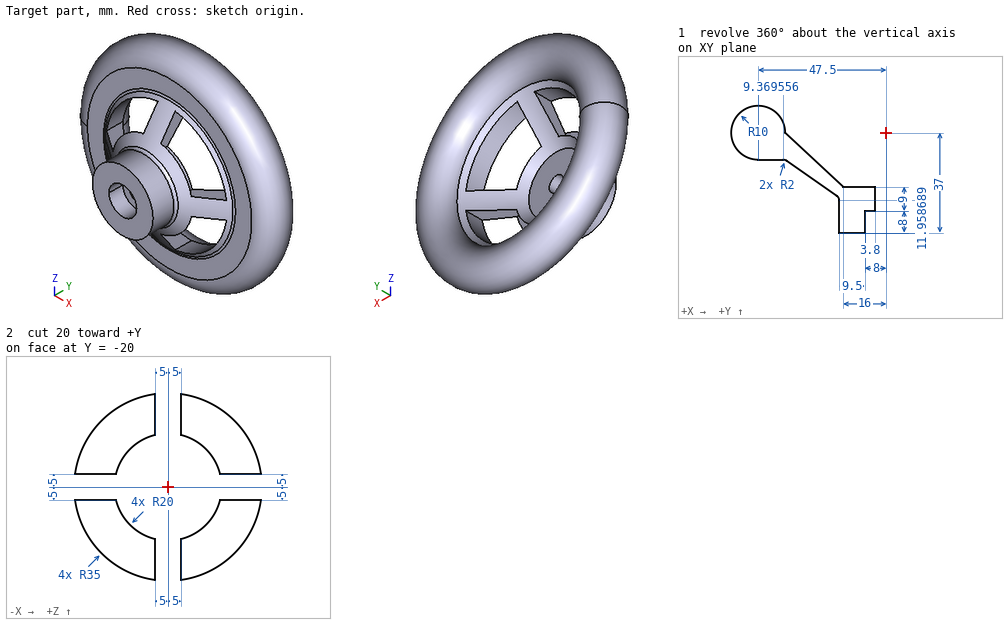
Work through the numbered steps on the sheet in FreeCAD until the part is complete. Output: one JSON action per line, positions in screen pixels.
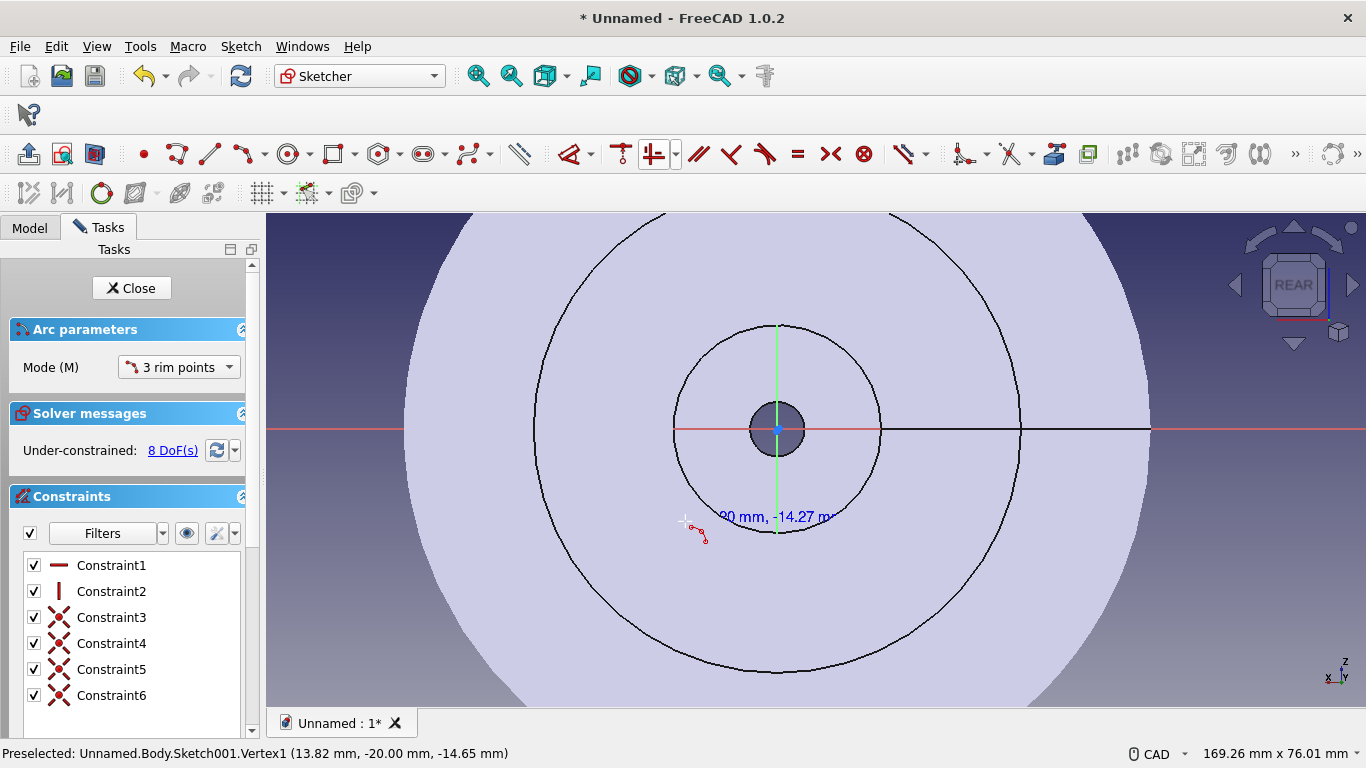
{"action": "left_click", "coordinate": [210, 154]}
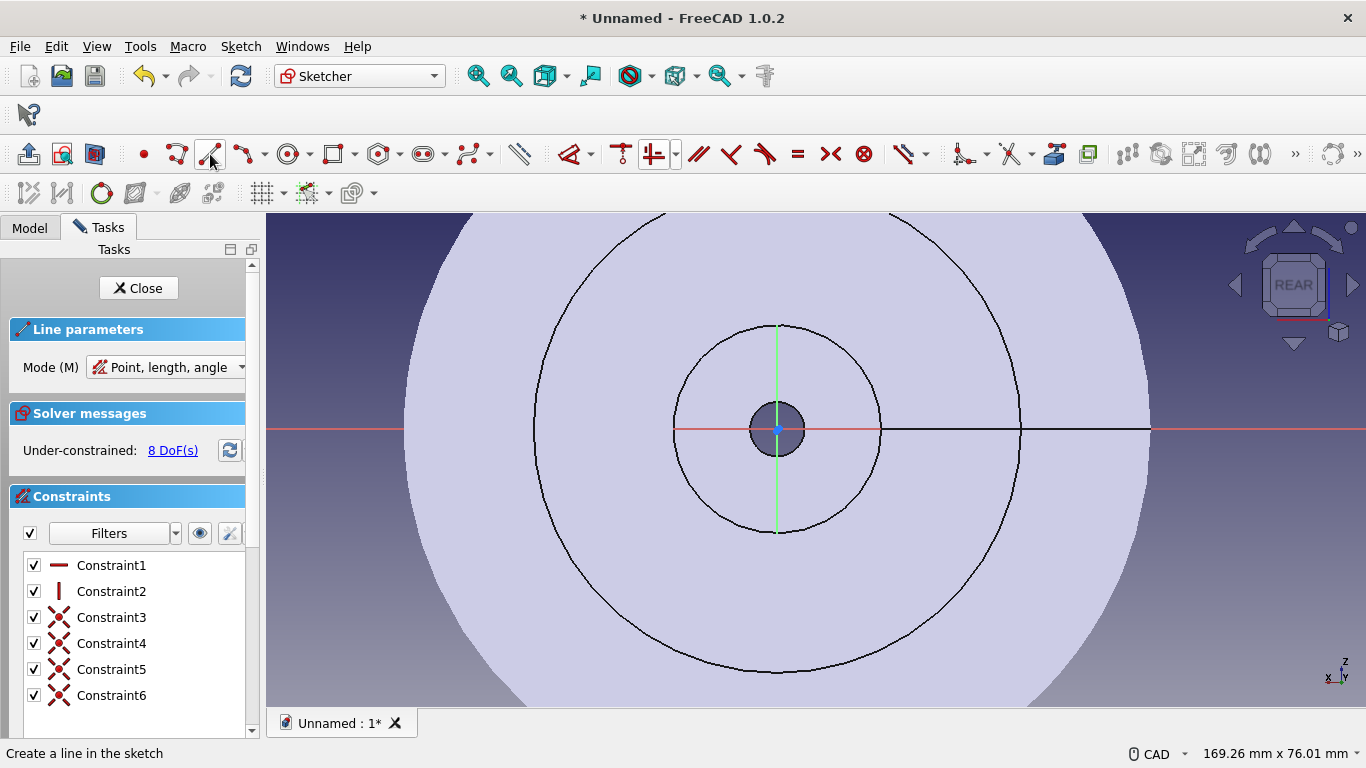
{"action": "left_click", "coordinate": [552, 397]}
{"action": "left_click", "coordinate": [651, 397]}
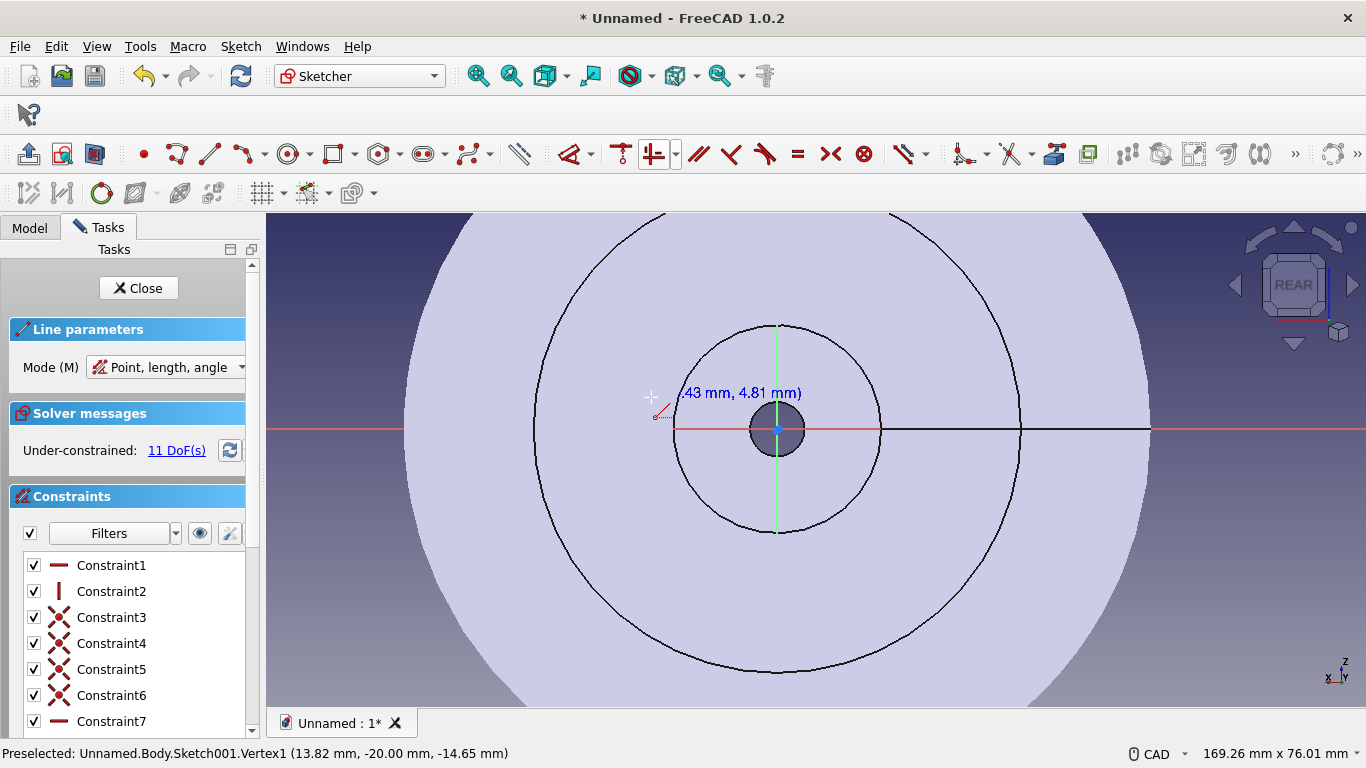
{"action": "left_click", "coordinate": [745, 303]}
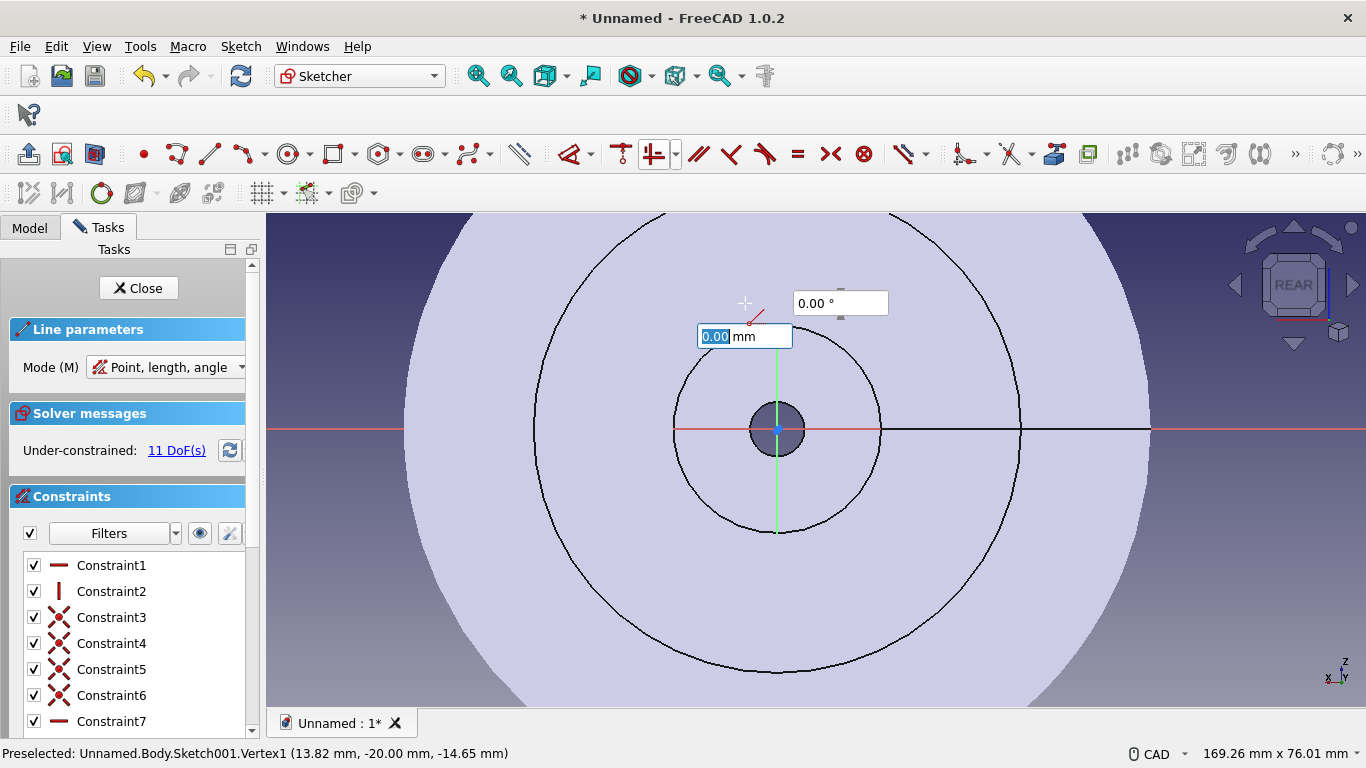
{"action": "scroll", "coordinate": [687, 523], "scroll_direction": "down", "scroll_amount": 2}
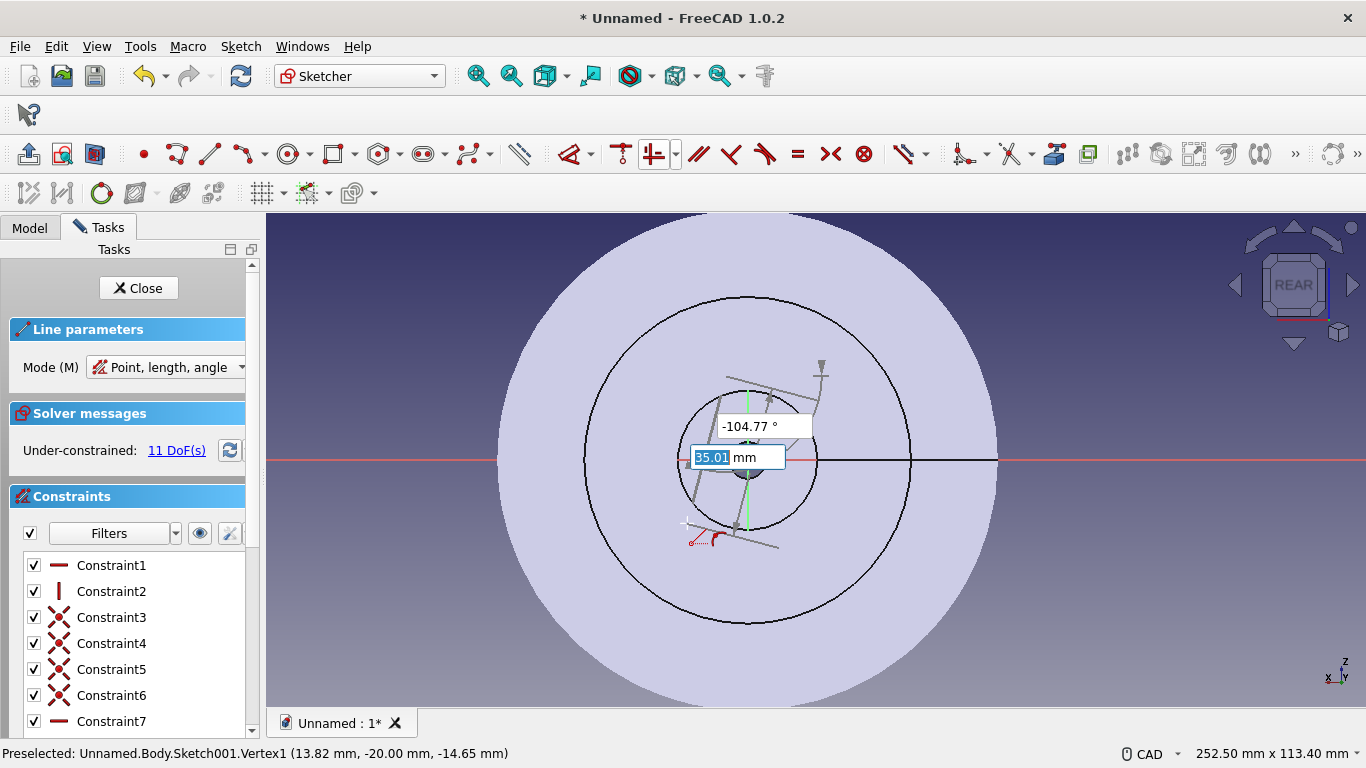
{"action": "left_click", "coordinate": [726, 309]}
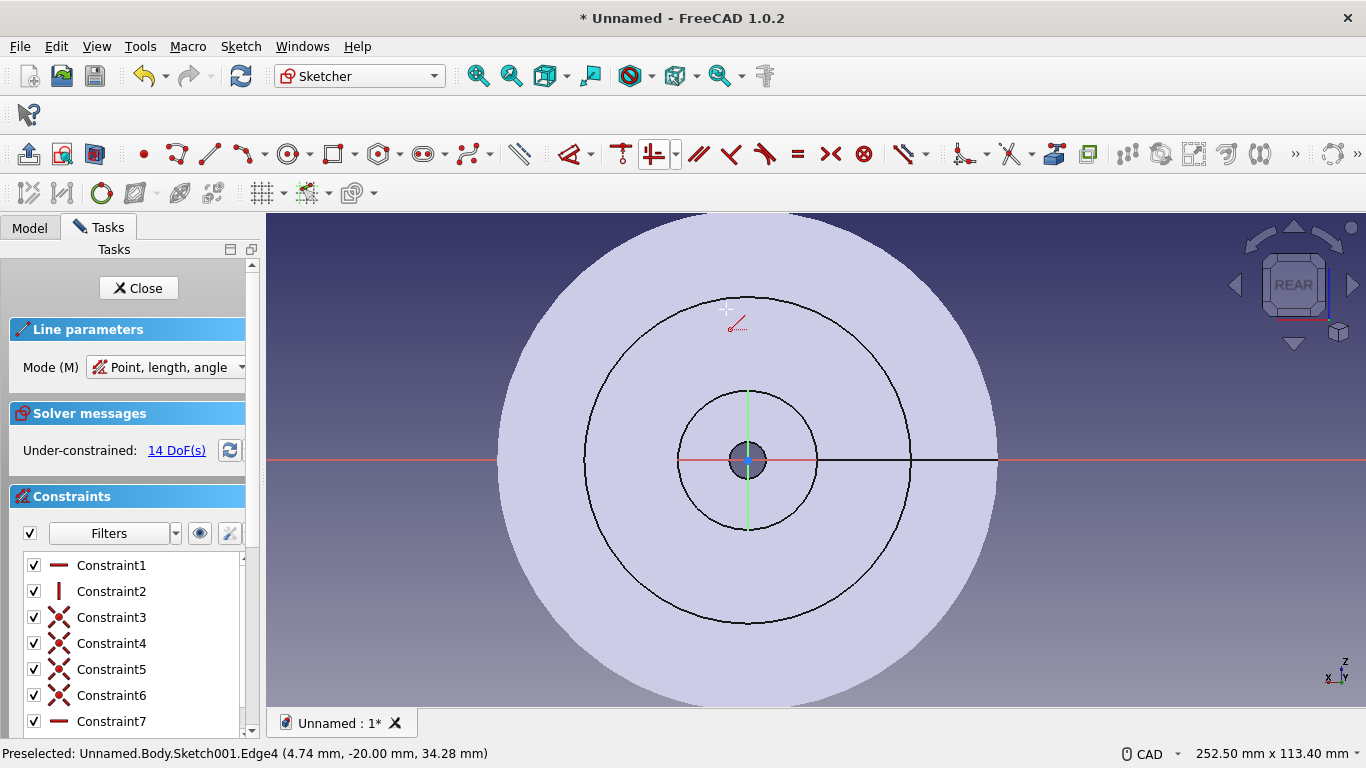
{"action": "left_click", "coordinate": [242, 154]}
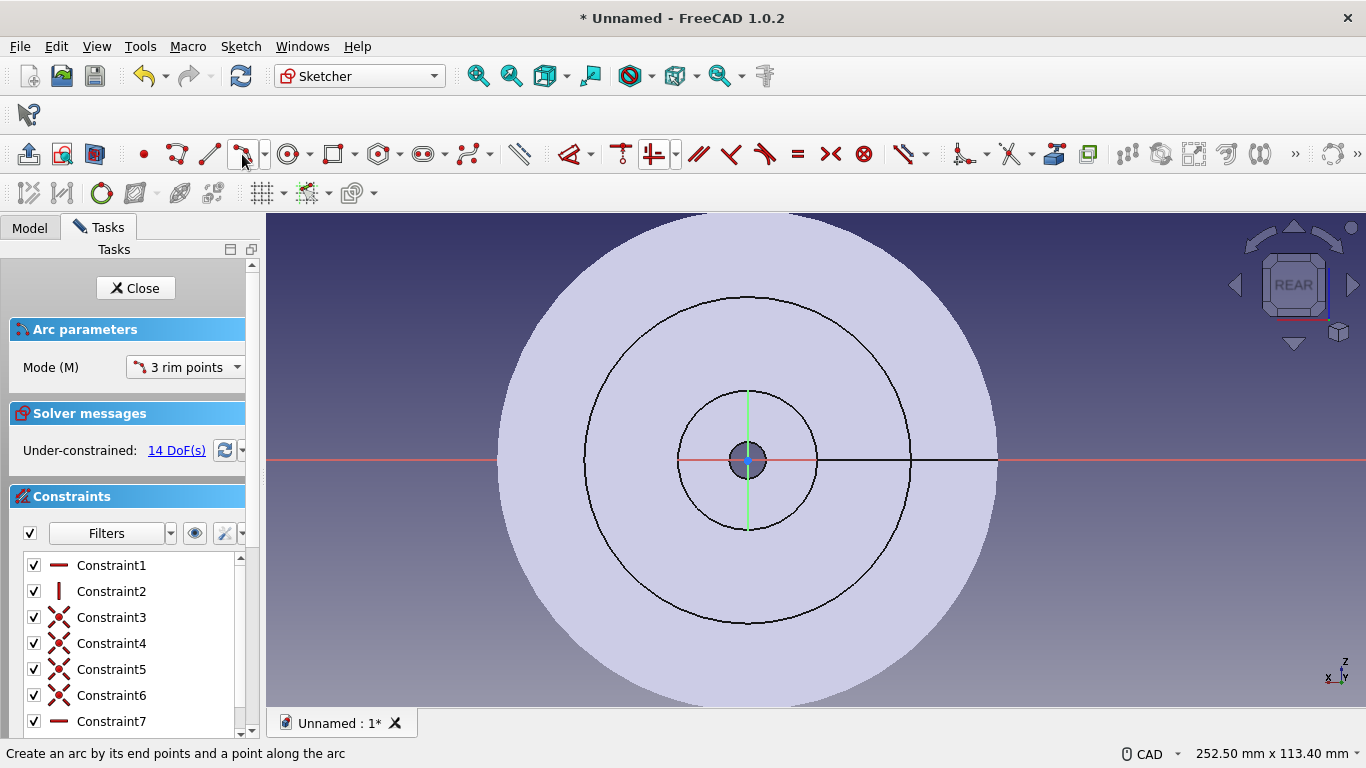
{"action": "left_click", "coordinate": [663, 439]}
{"action": "left_click", "coordinate": [726, 376]}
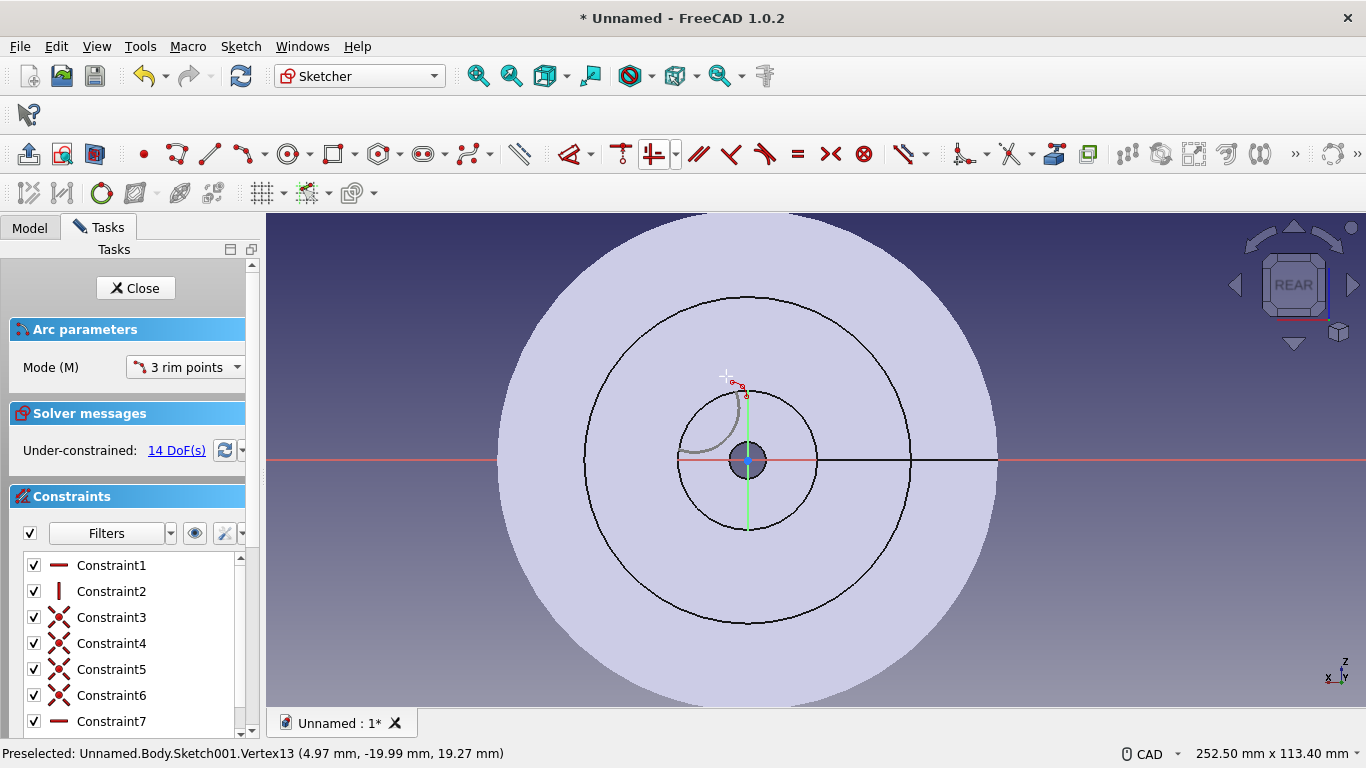
{"action": "scroll", "coordinate": [686, 399], "scroll_direction": "up", "scroll_amount": 2}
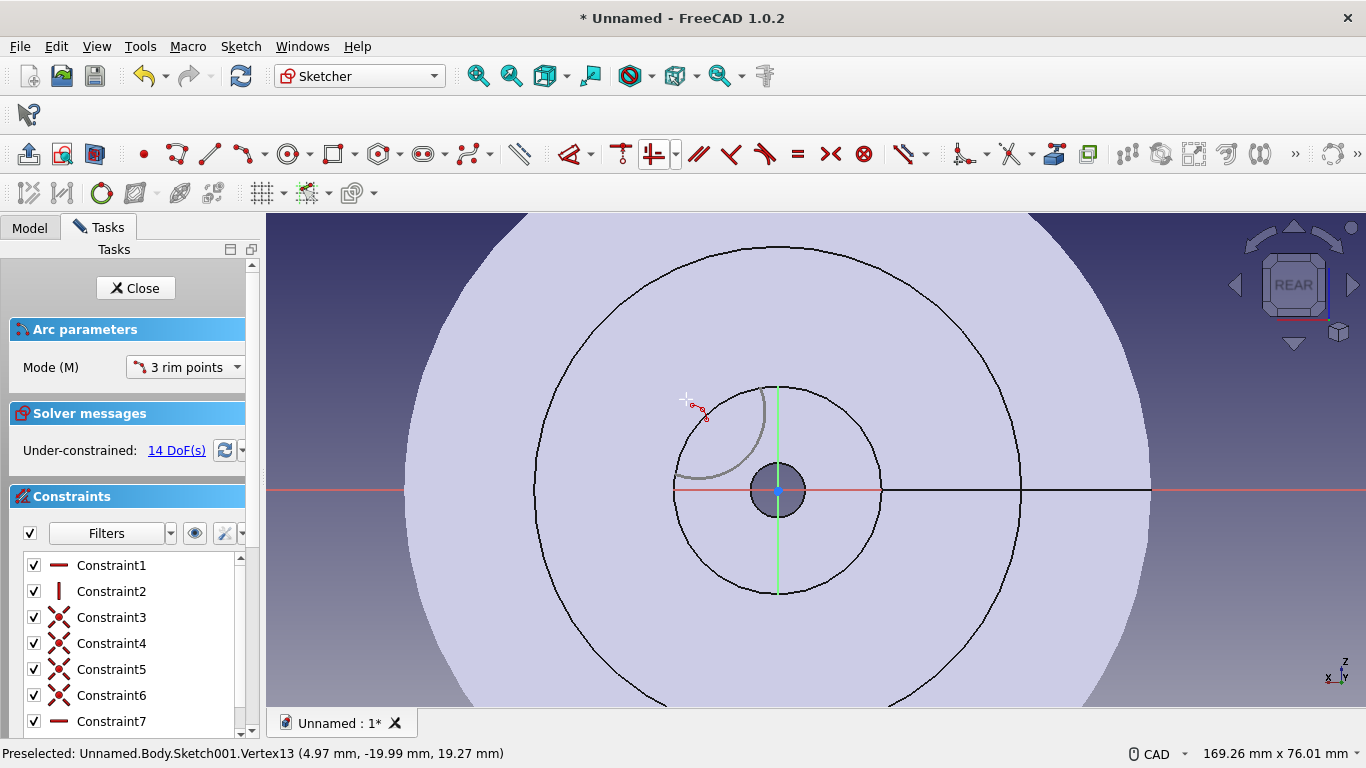
{"action": "left_click", "coordinate": [686, 398]}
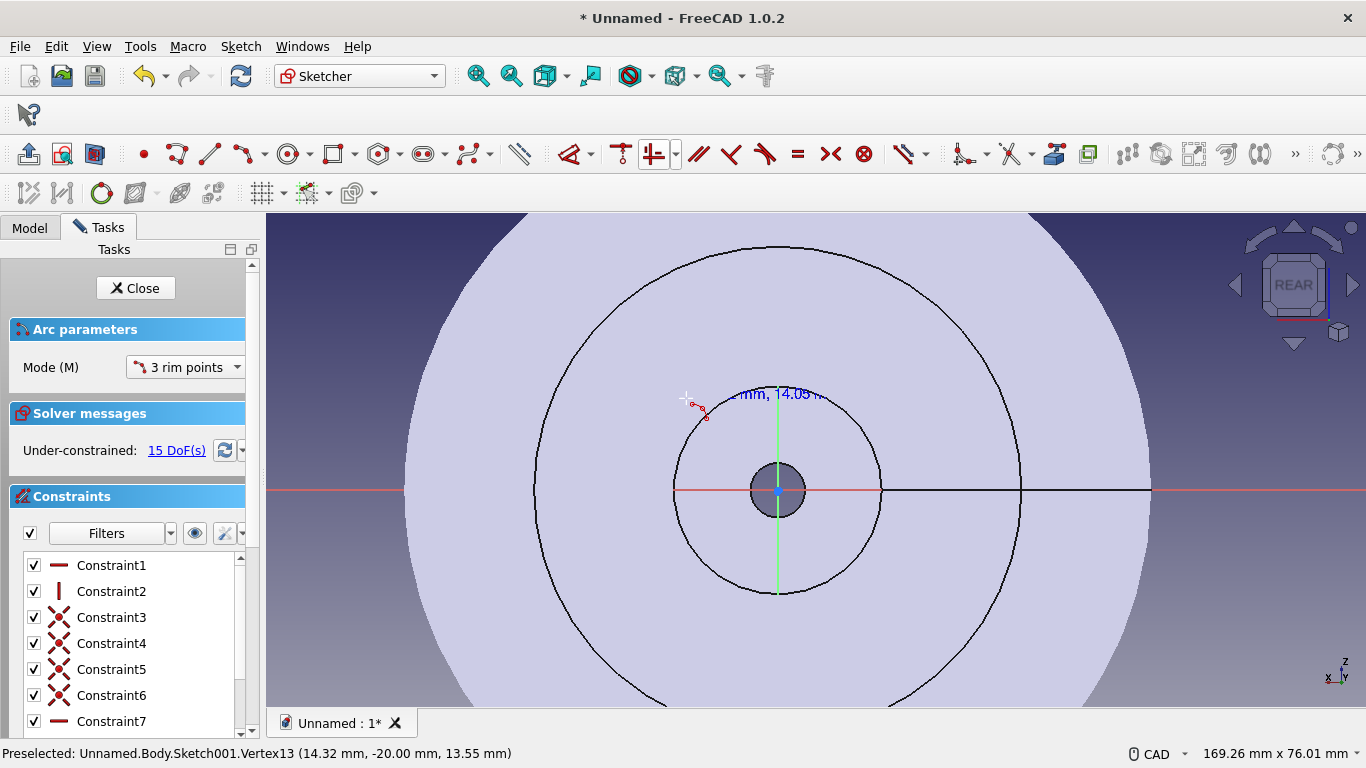
{"action": "left_click", "coordinate": [745, 266]}
{"action": "left_click", "coordinate": [552, 459]}
{"action": "left_click", "coordinate": [617, 329]}